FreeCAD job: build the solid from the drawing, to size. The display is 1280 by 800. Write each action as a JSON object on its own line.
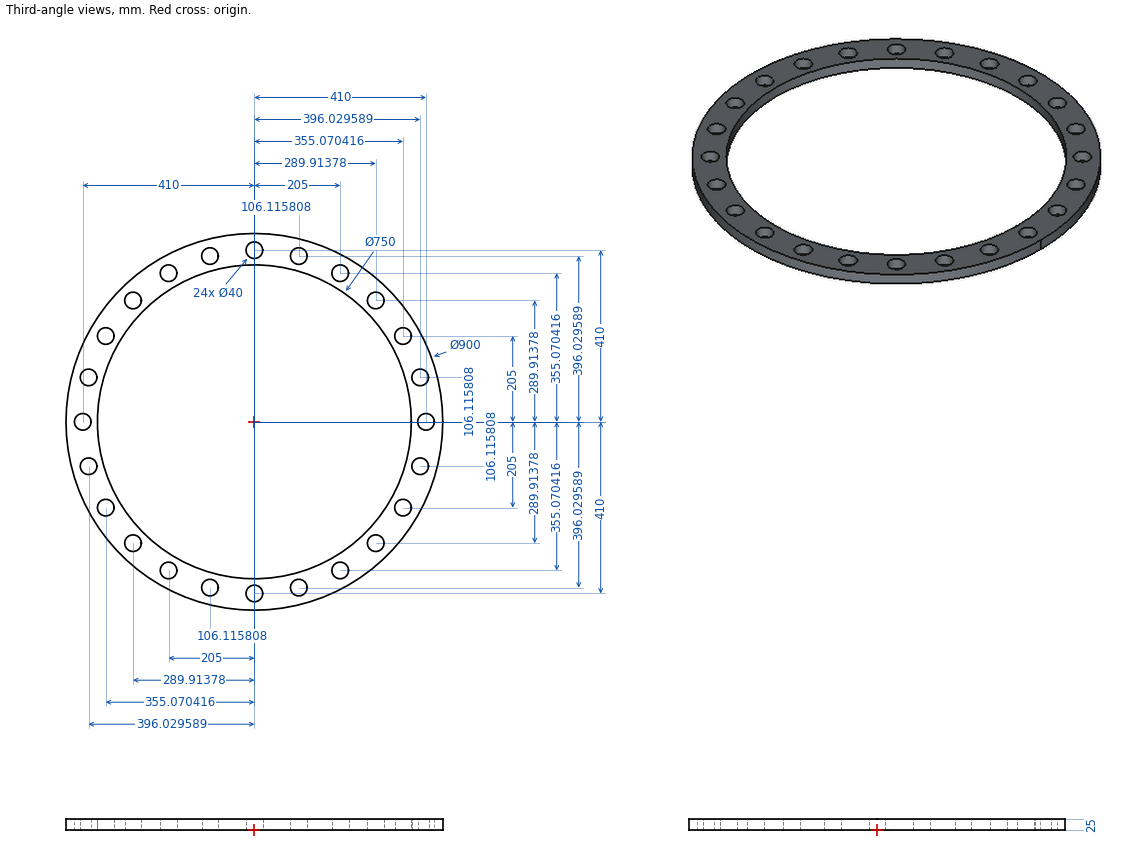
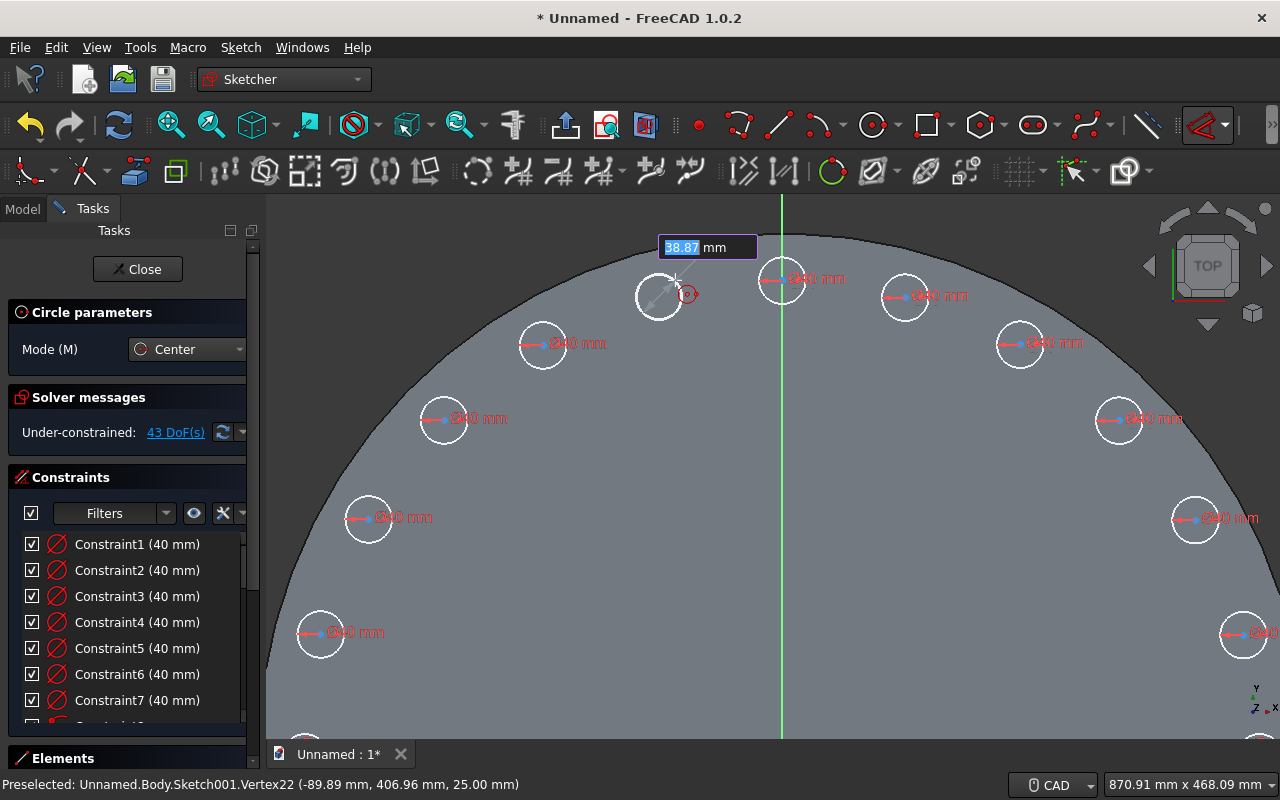
{"action": "type", "text": "40"}
{"action": "key", "text": "Return"}
{"action": "key", "text": "Escape"}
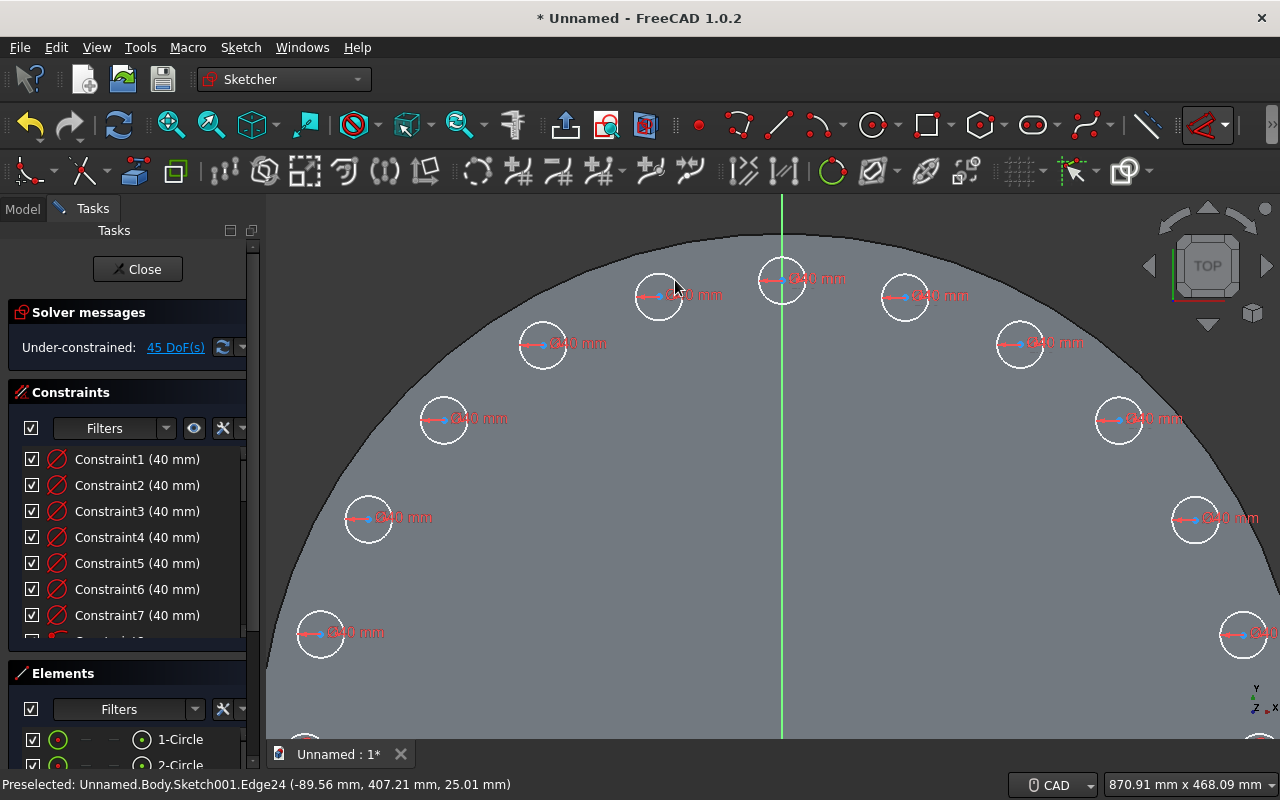
{"action": "left_click", "coordinate": [782, 281]}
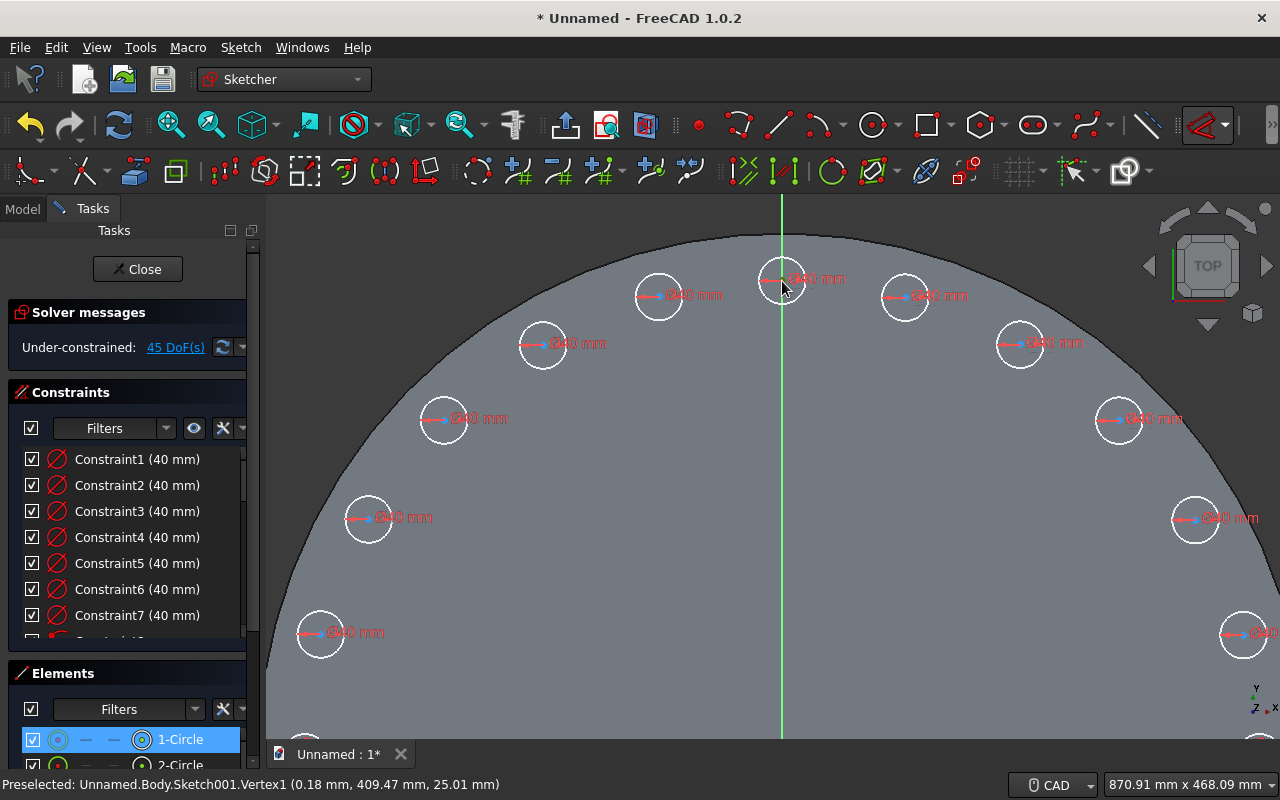
{"action": "left_click", "coordinate": [782, 676]}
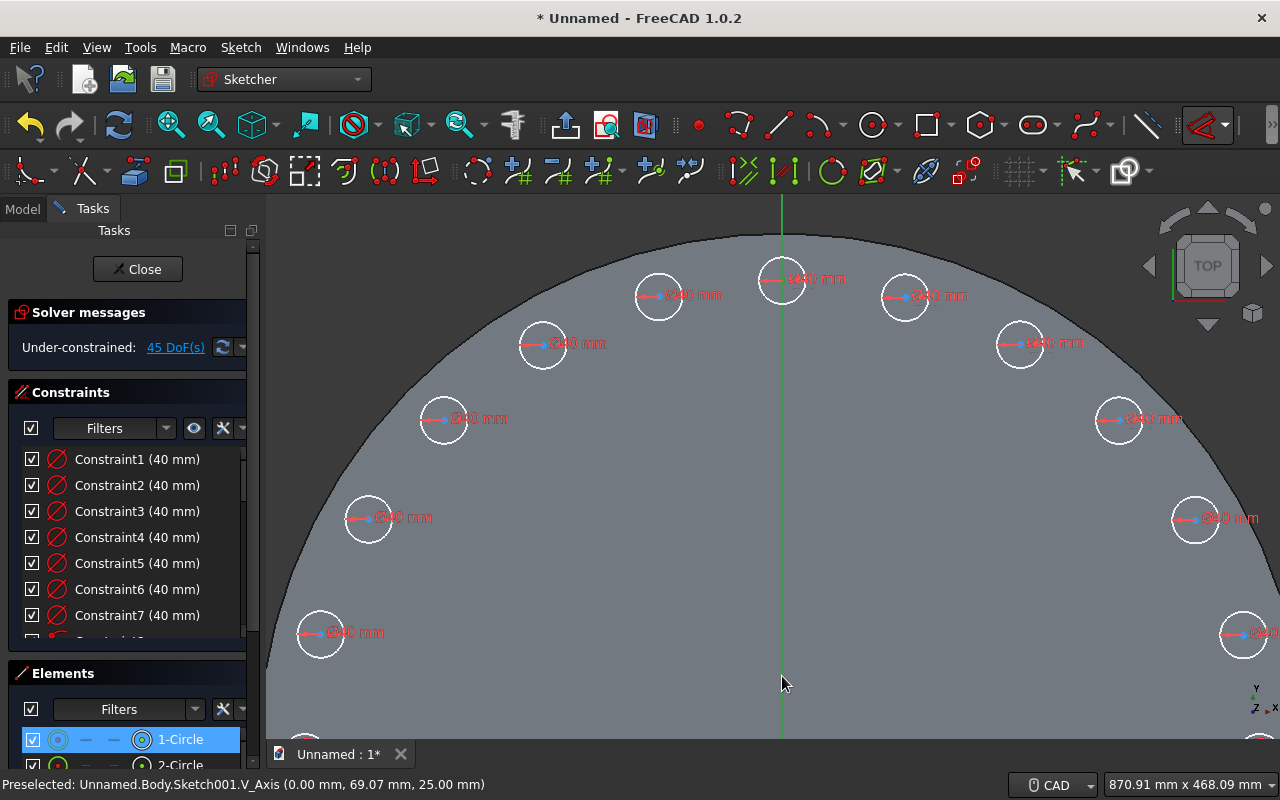
{"action": "key", "text": "c"}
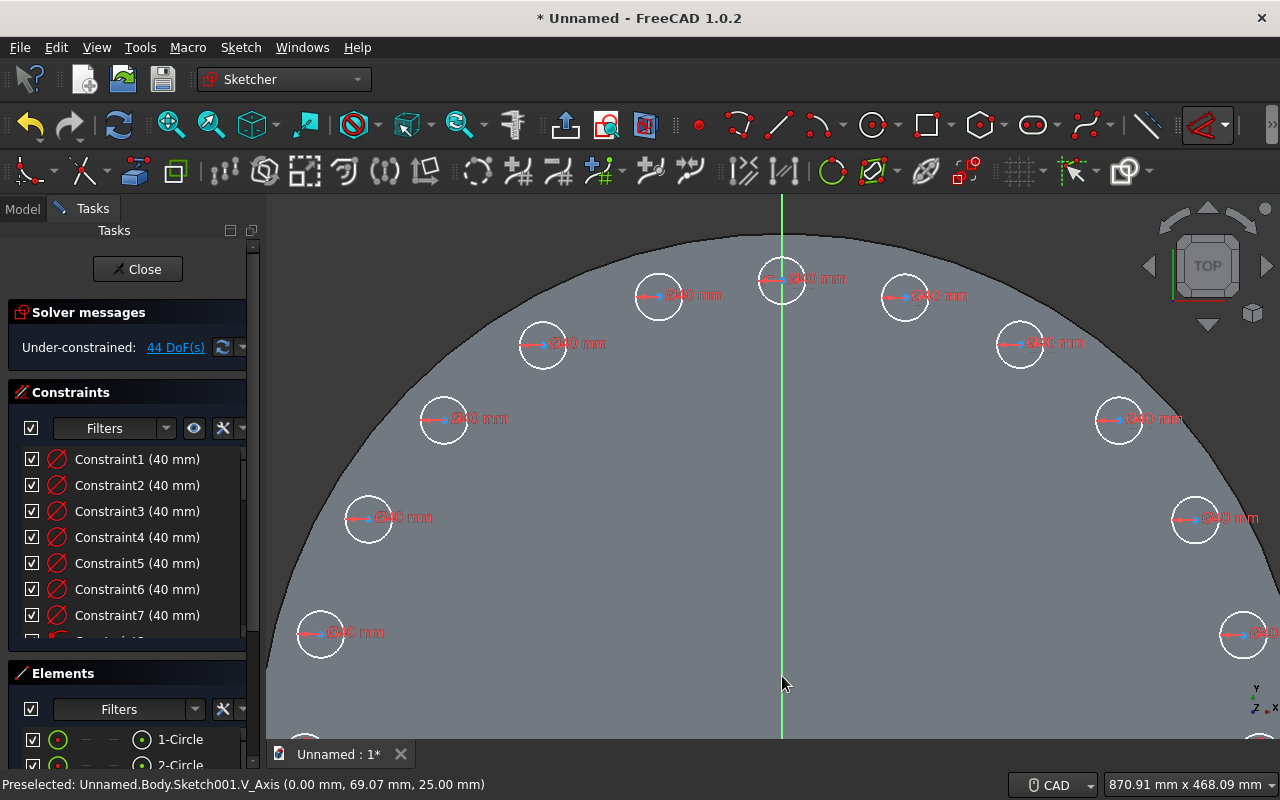
{"action": "scroll", "coordinate": [659, 297], "scroll_direction": "down", "scroll_amount": 5}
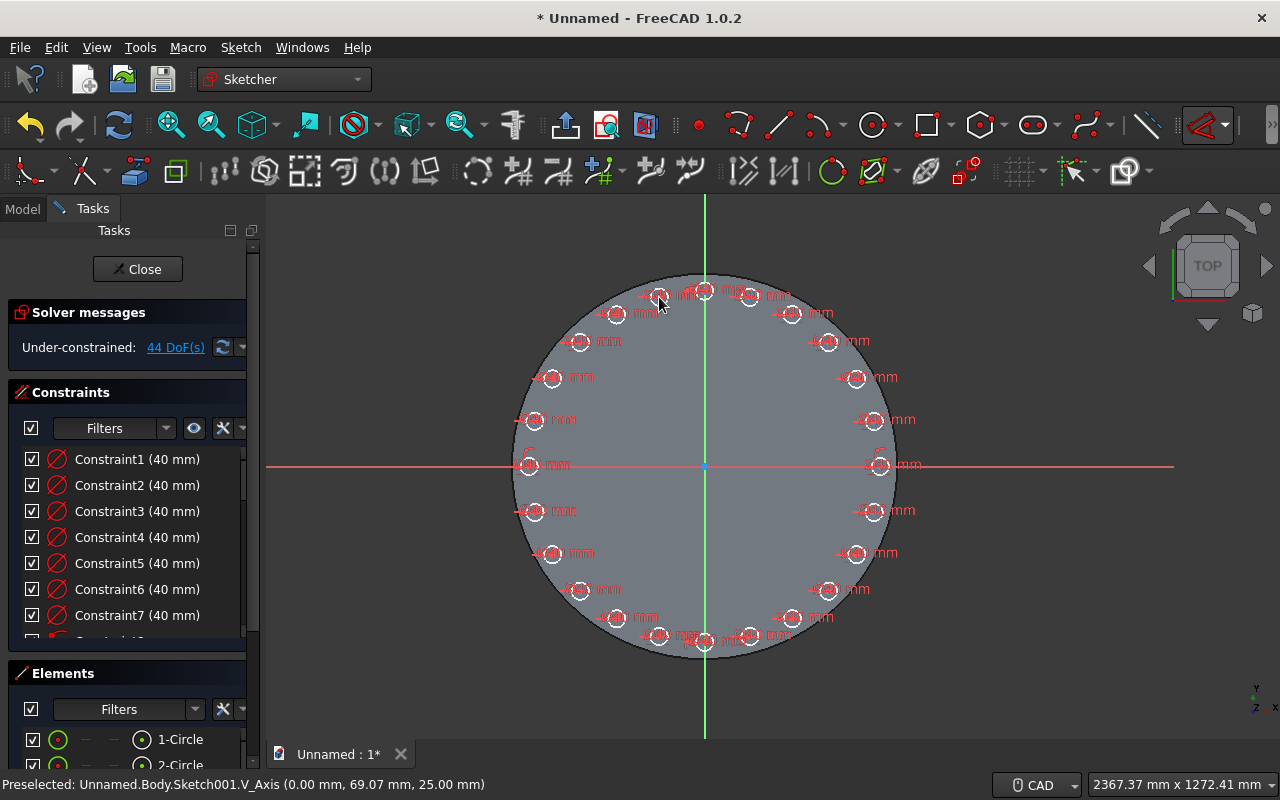
{"action": "left_click", "coordinate": [874, 422]}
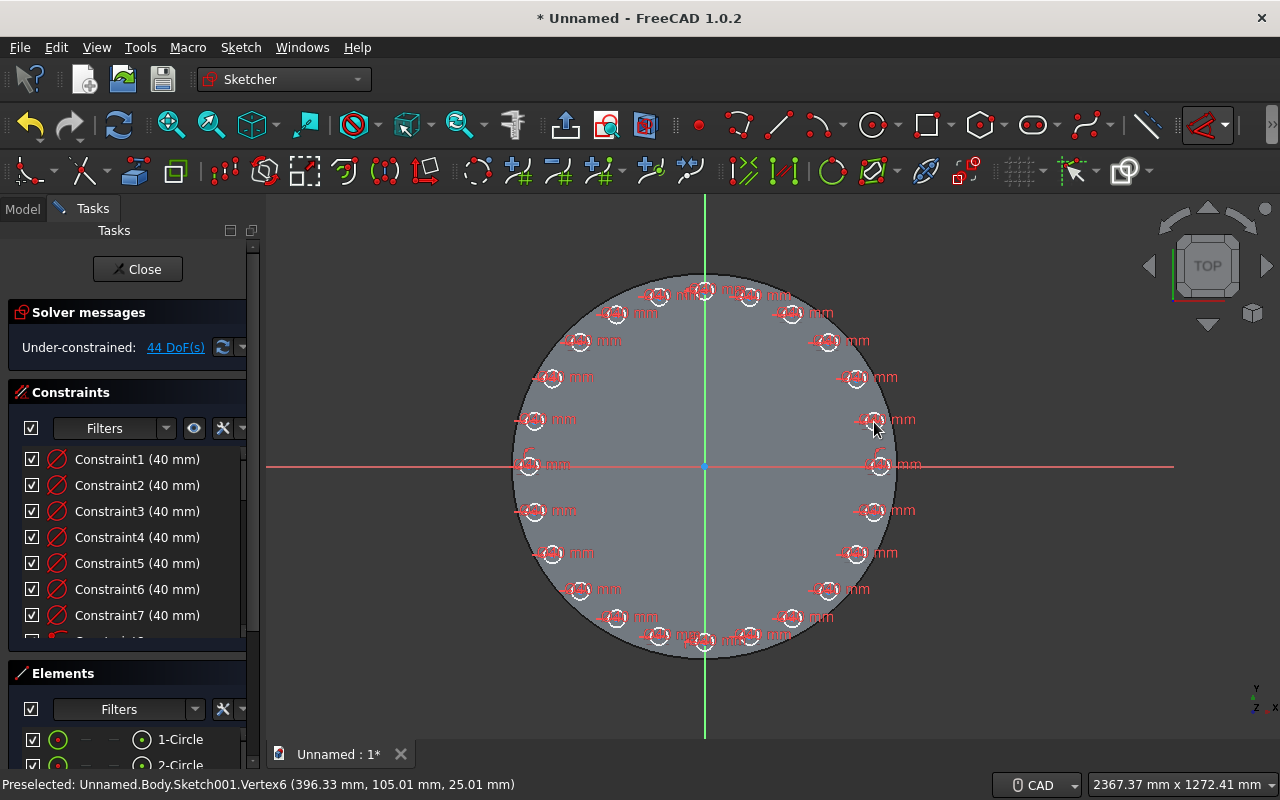
{"action": "left_click", "coordinate": [874, 512]}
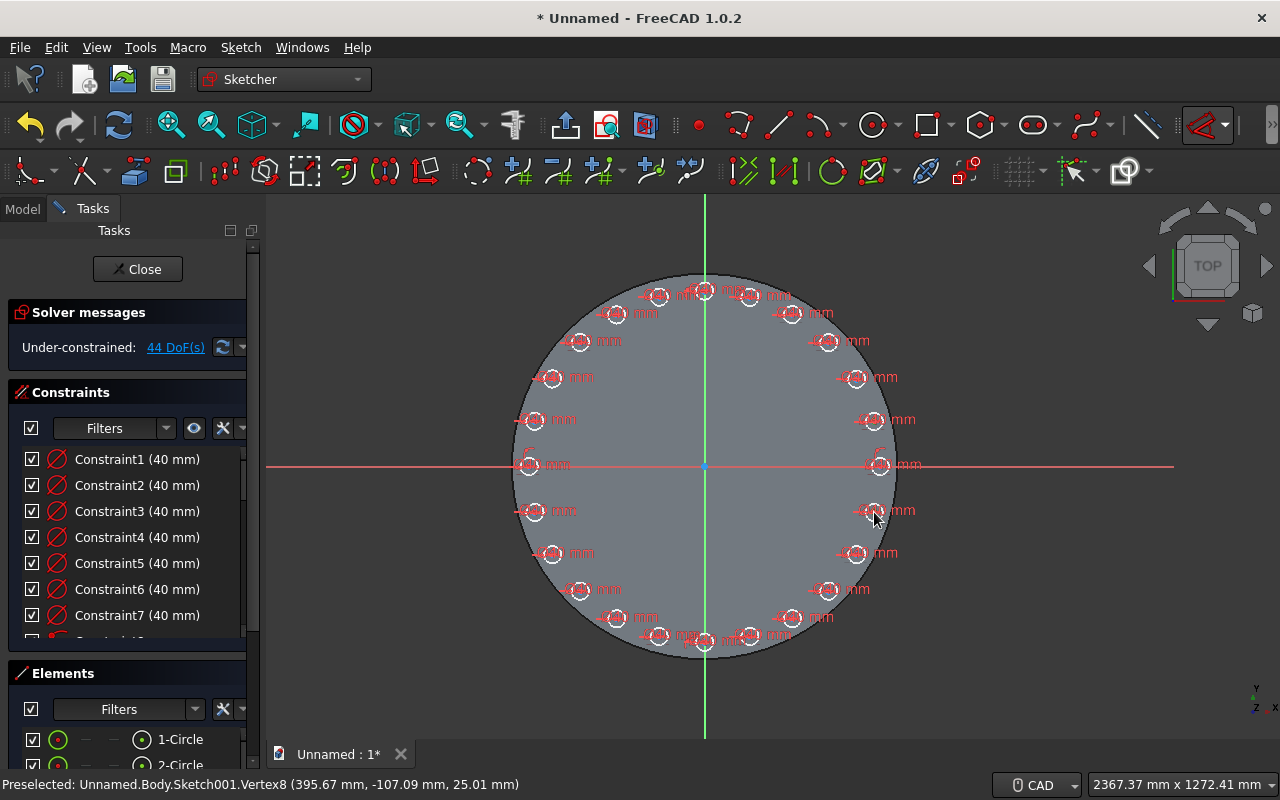
{"action": "key", "text": "v"}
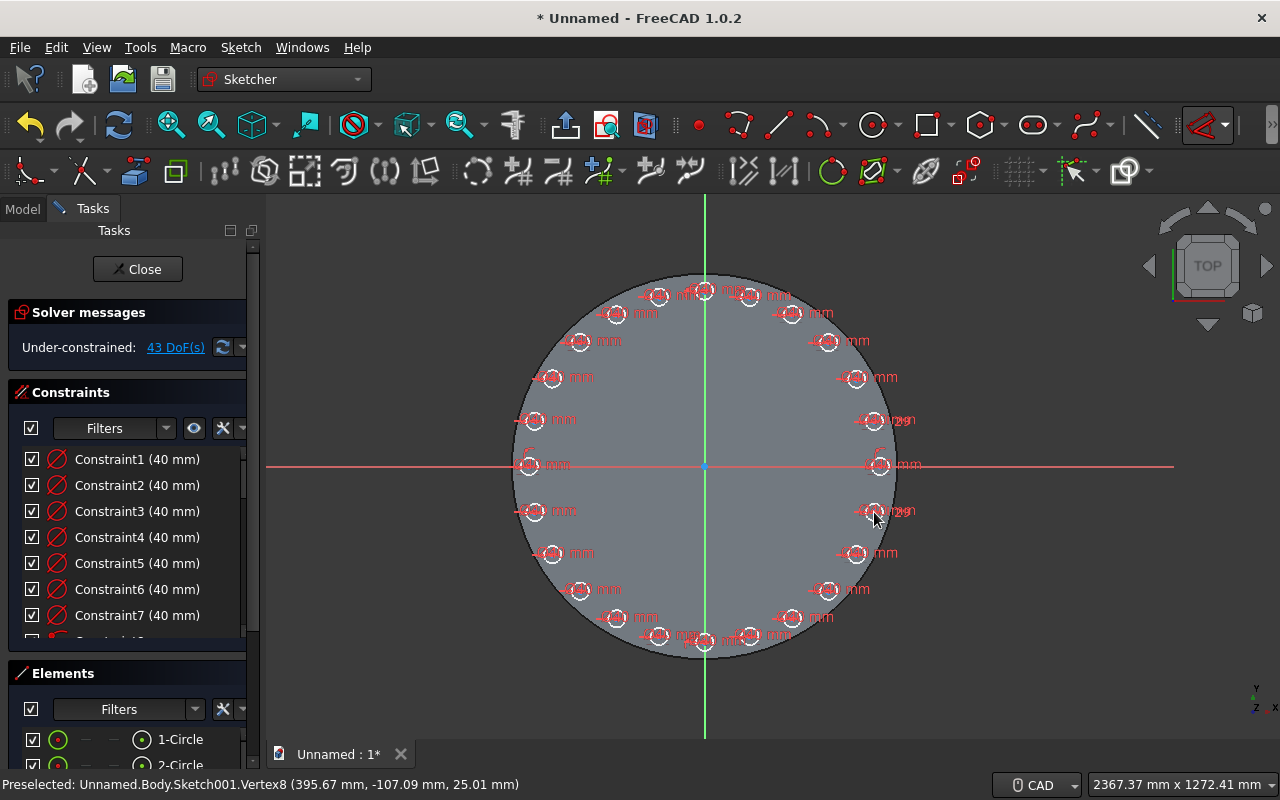
{"action": "left_click", "coordinate": [857, 379]}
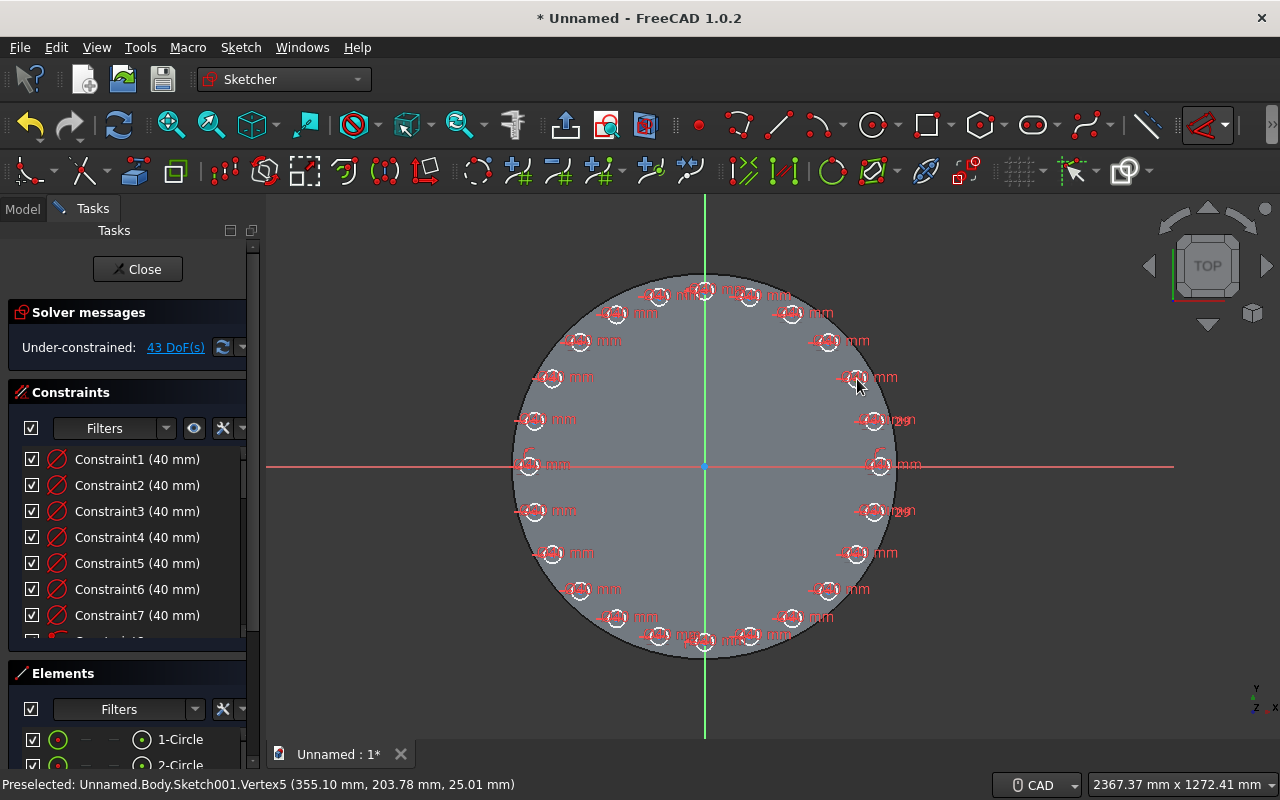
{"action": "left_click", "coordinate": [857, 555]}